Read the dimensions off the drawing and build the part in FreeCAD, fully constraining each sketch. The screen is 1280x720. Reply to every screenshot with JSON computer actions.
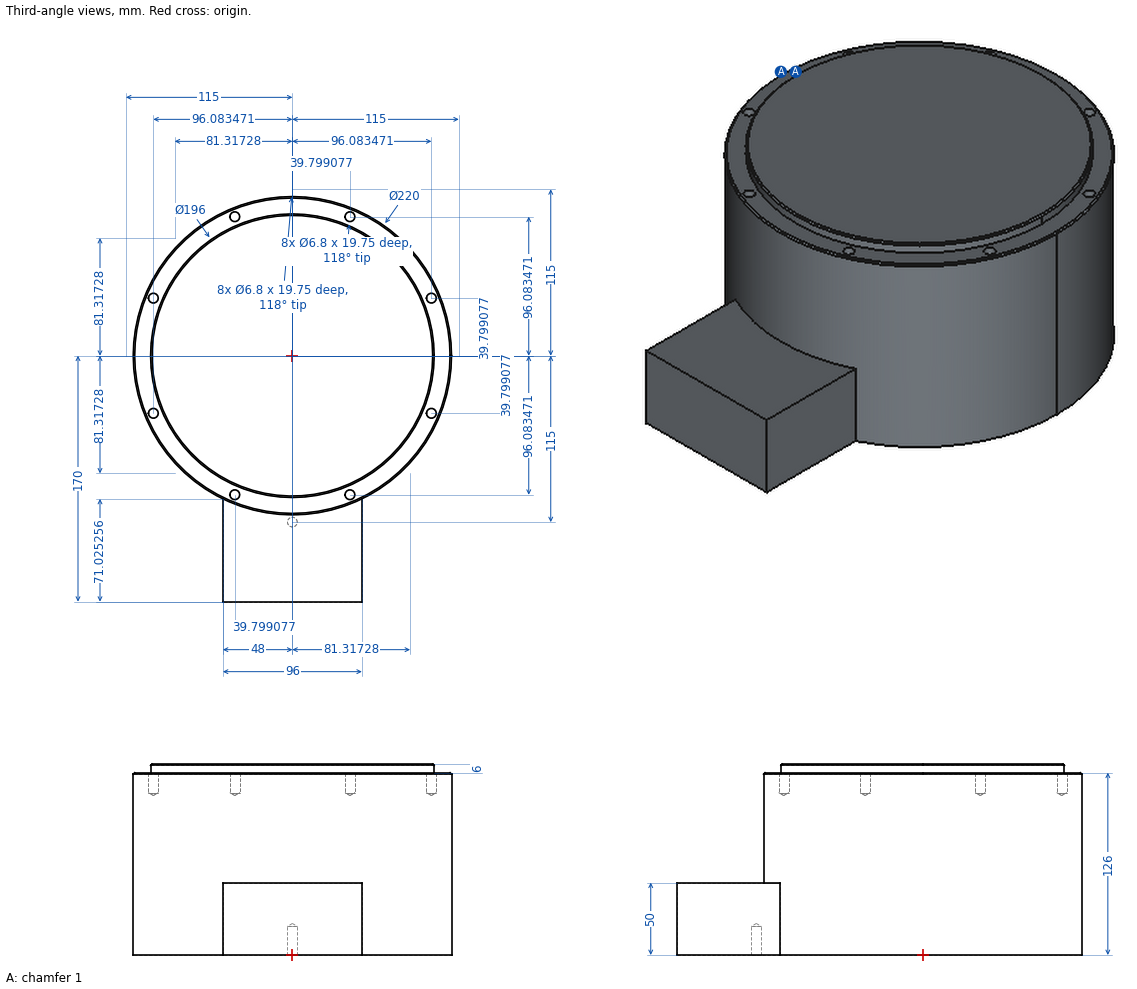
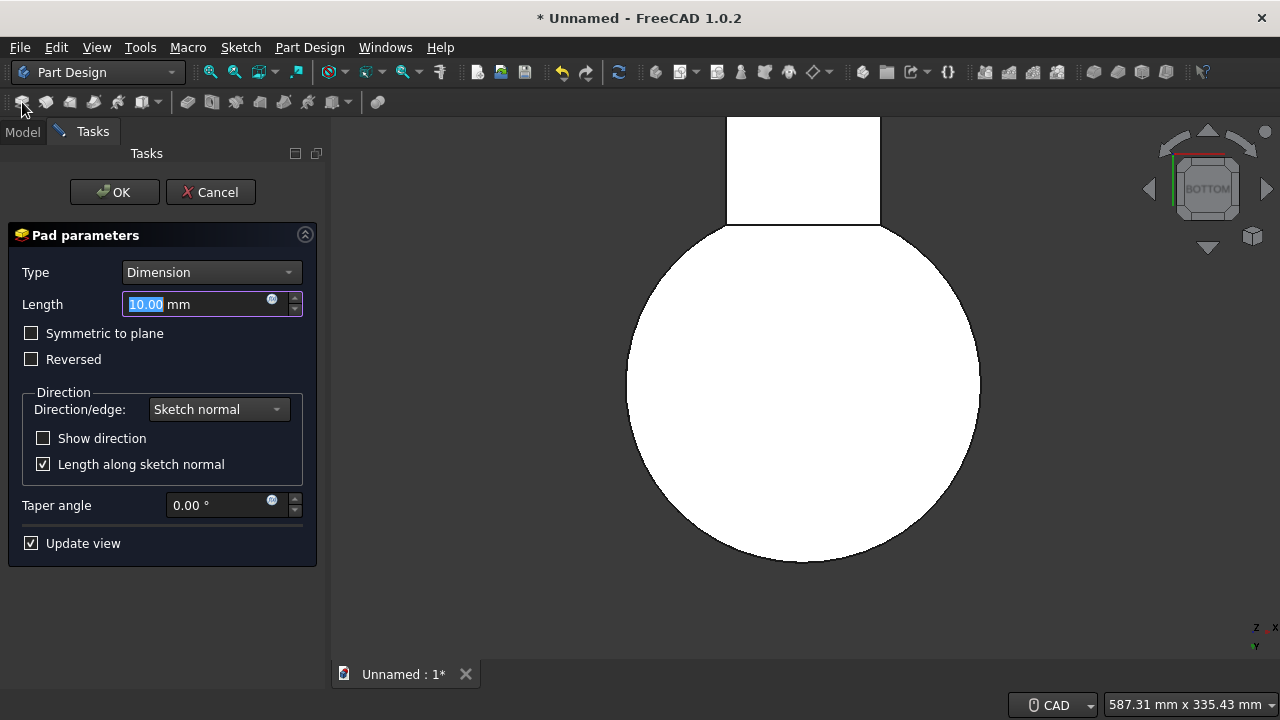
{"action": "type", "text": "50"}
{"action": "key", "text": "Tab"}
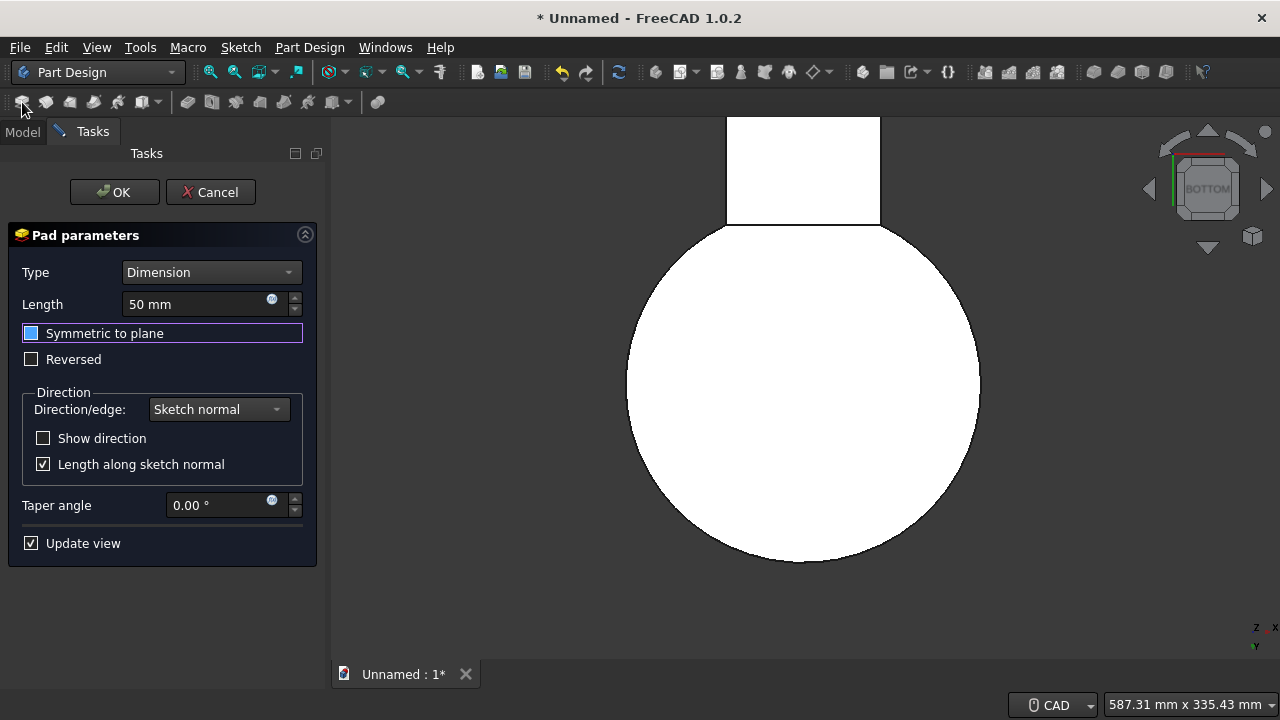
{"action": "left_click", "coordinate": [30, 359]}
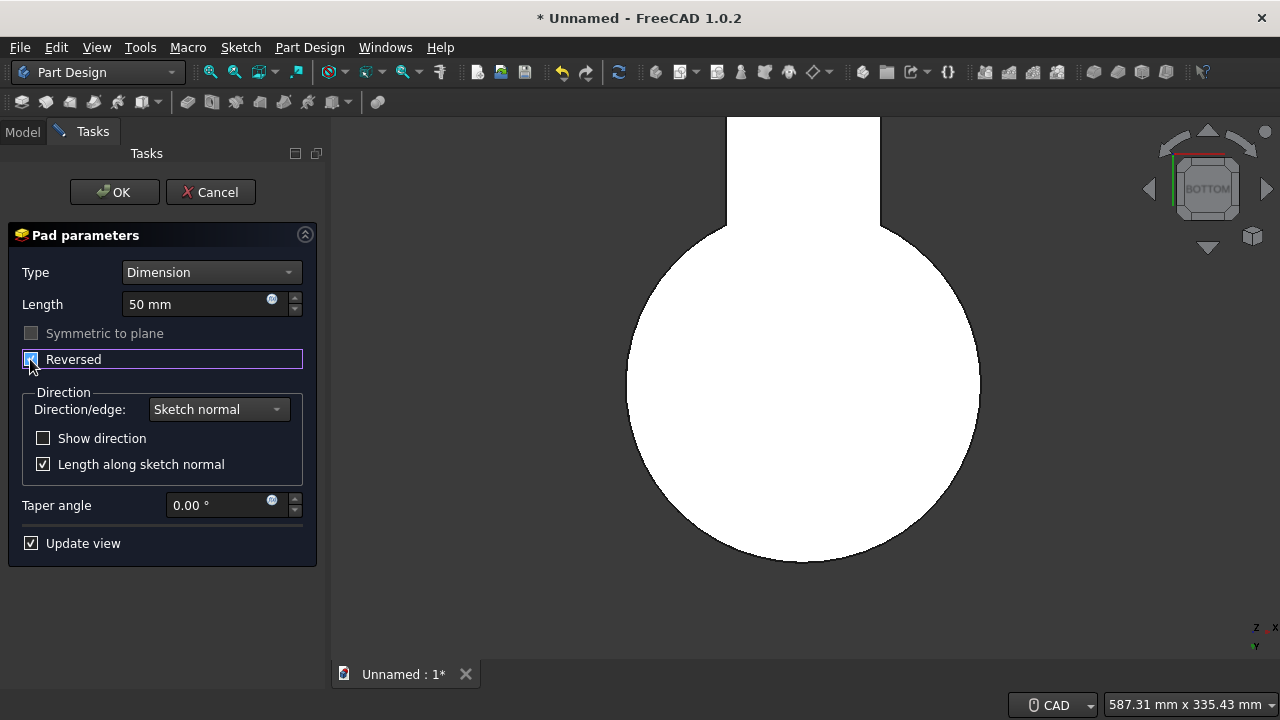
{"action": "left_click", "coordinate": [115, 192]}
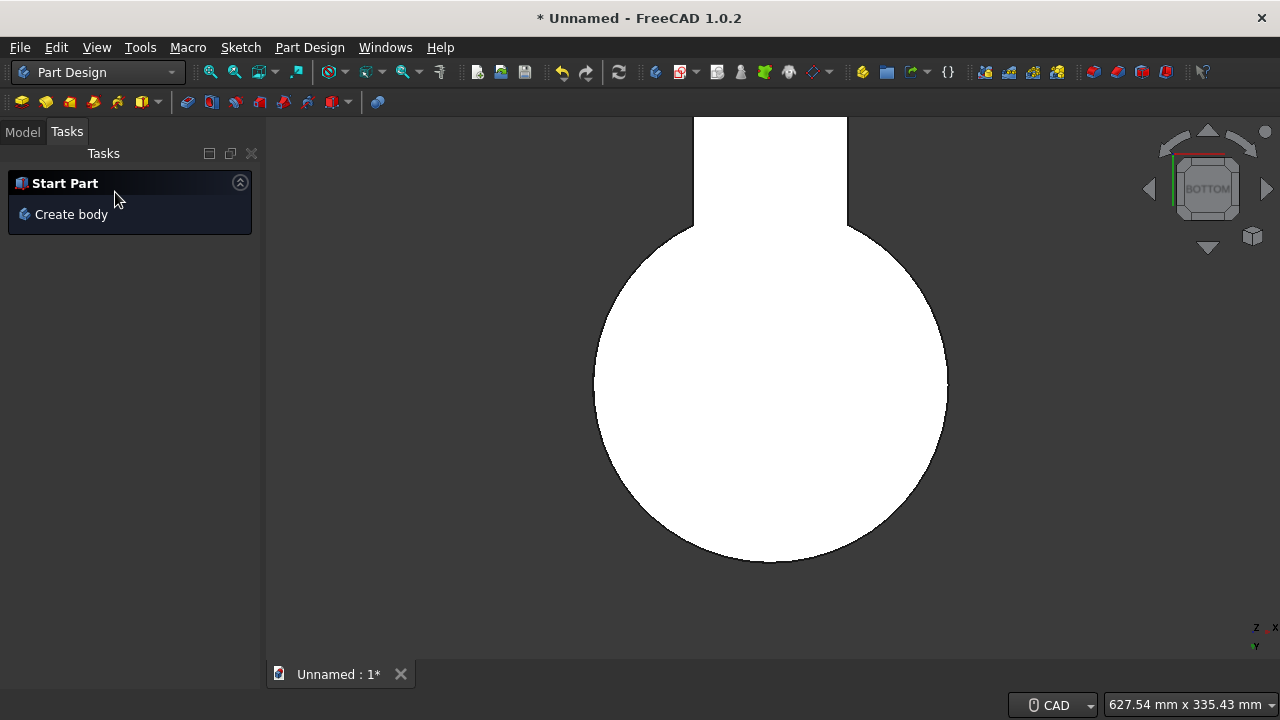
{"action": "left_click", "coordinate": [212, 72]}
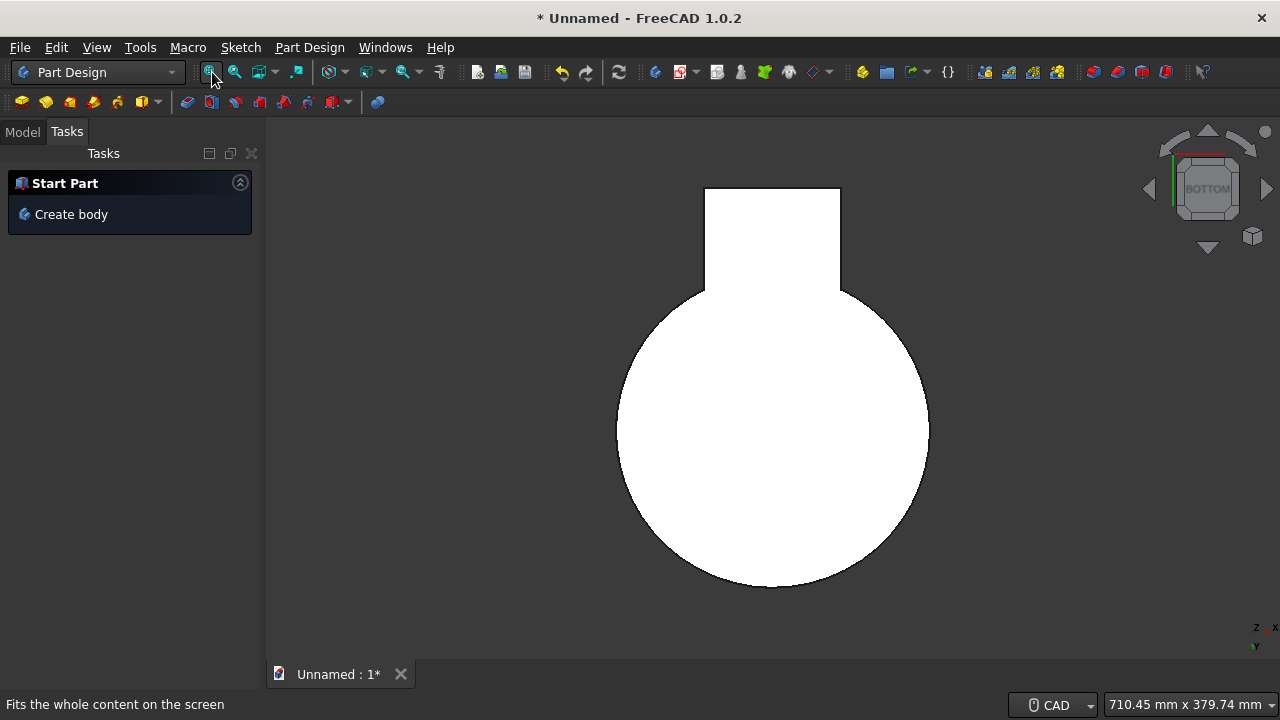
{"action": "key", "text": "0"}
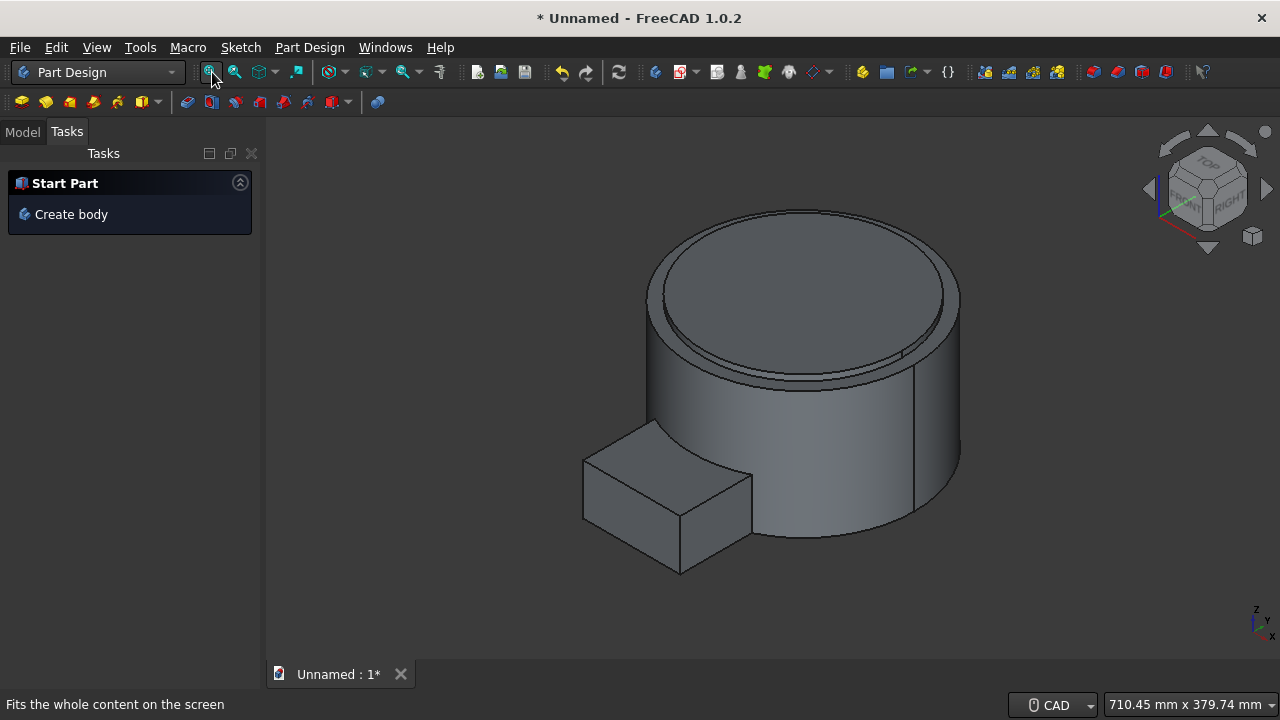
{"action": "left_click", "coordinate": [663, 341]}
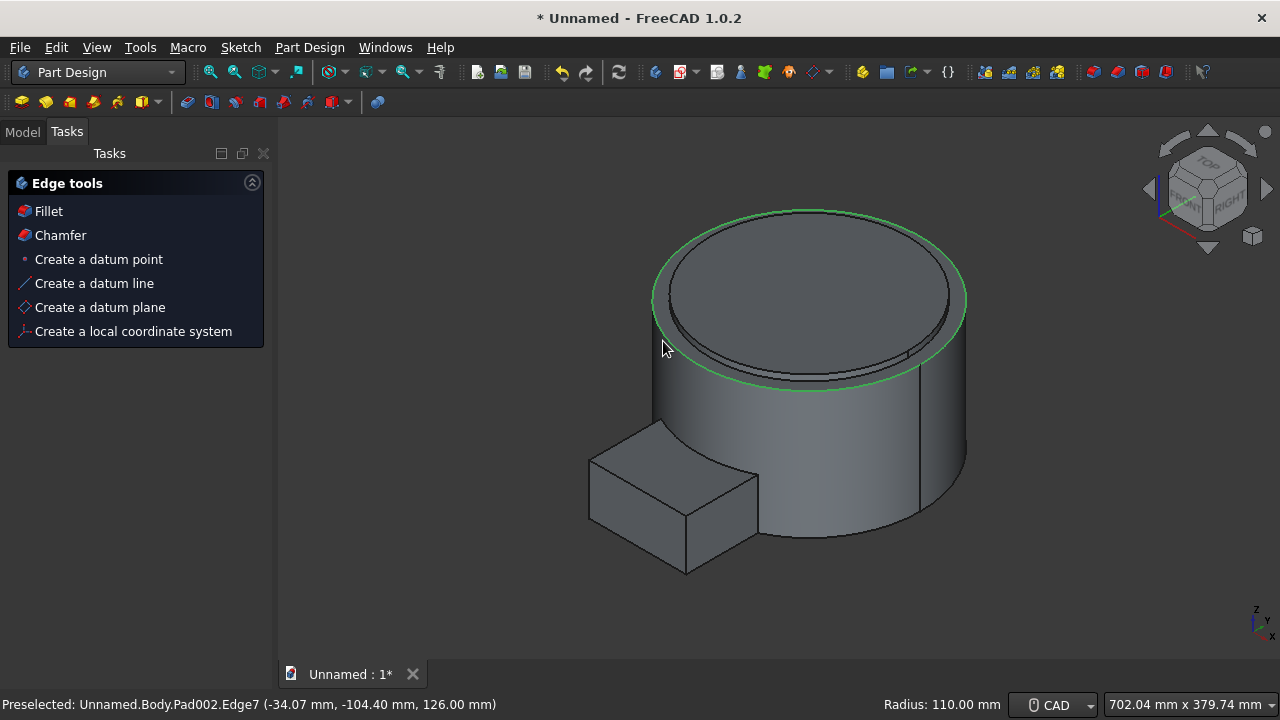
{"action": "left_click", "coordinate": [685, 329], "text": "ctrl"}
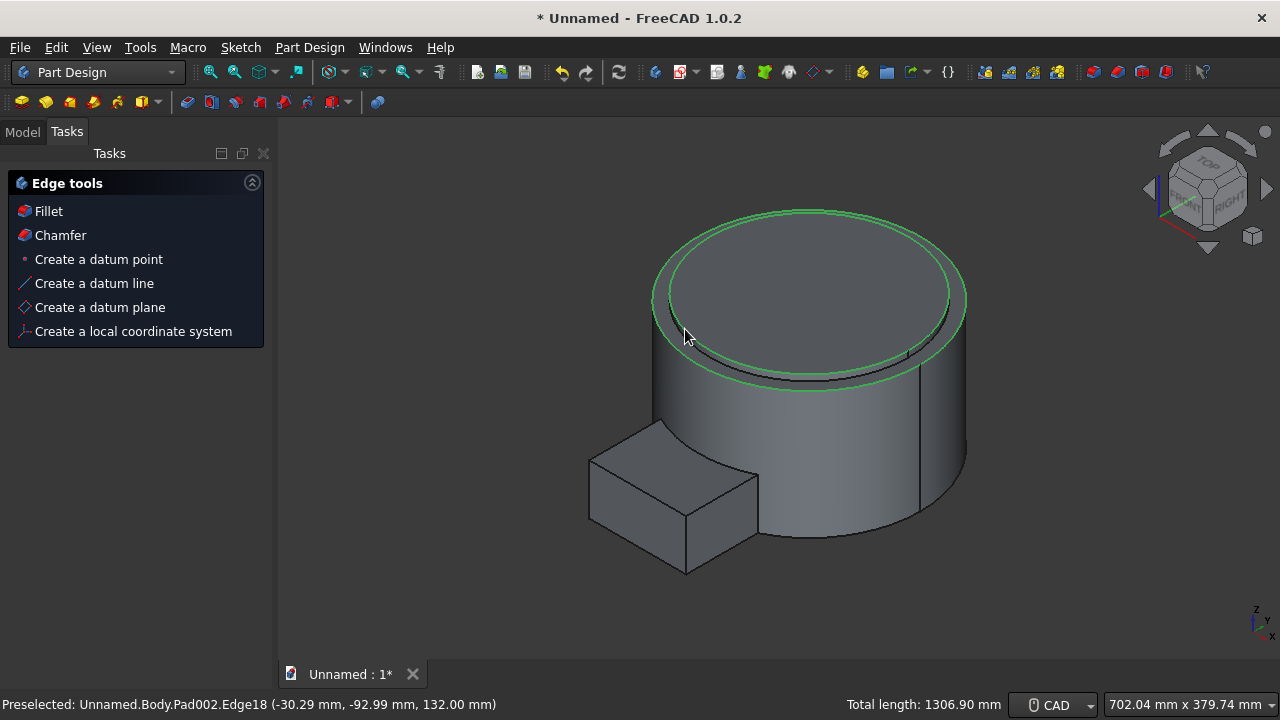
{"action": "left_click", "coordinate": [1118, 72]}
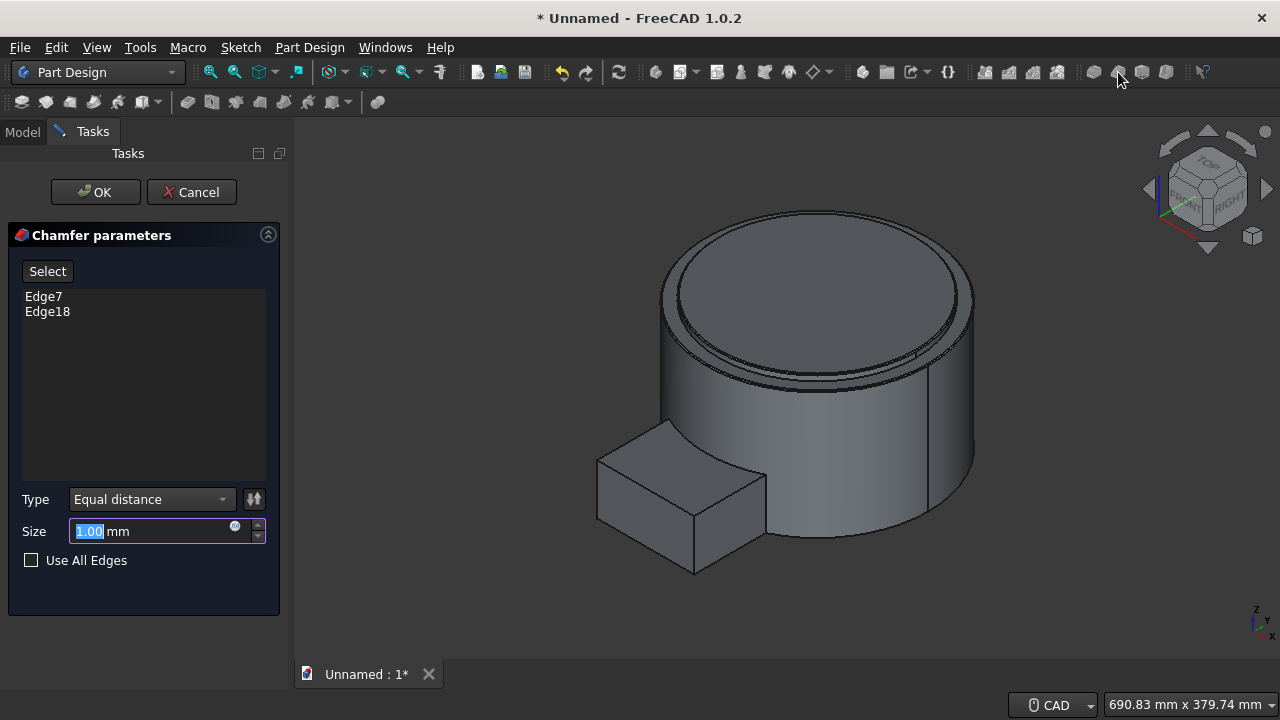
{"action": "type", "text": "1"}
{"action": "key", "text": "Tab"}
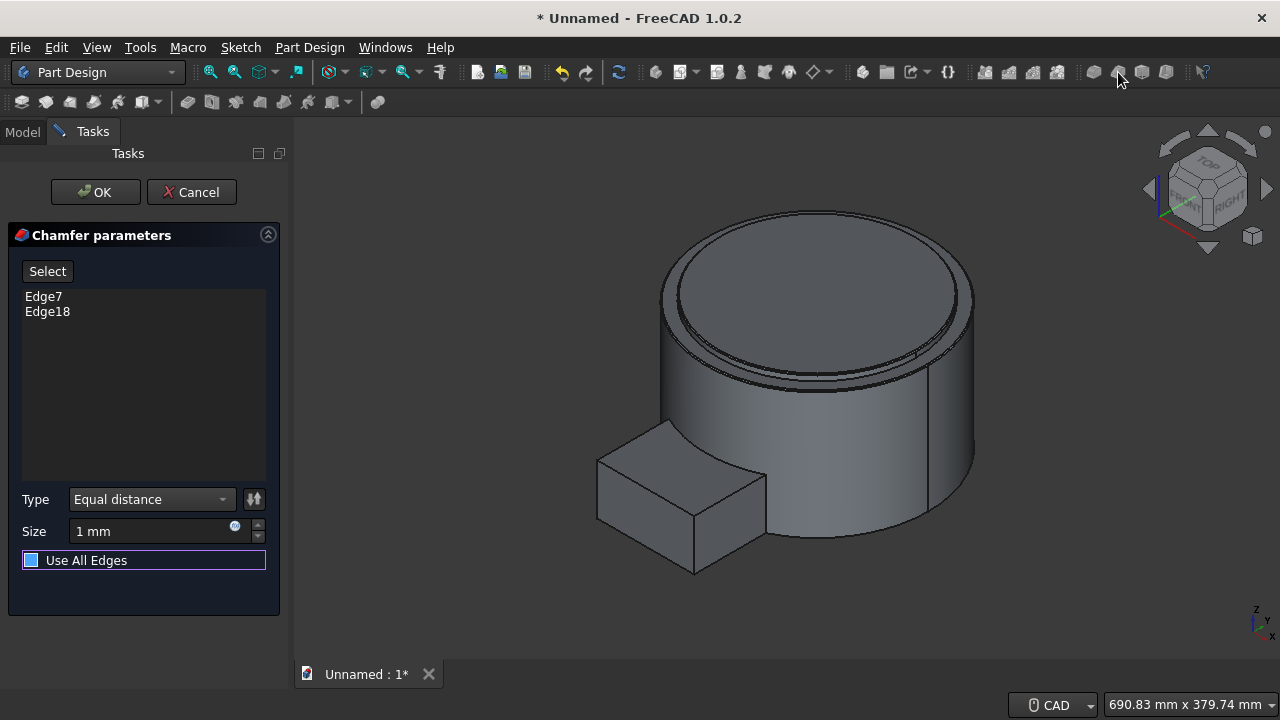
{"action": "left_click", "coordinate": [96, 192]}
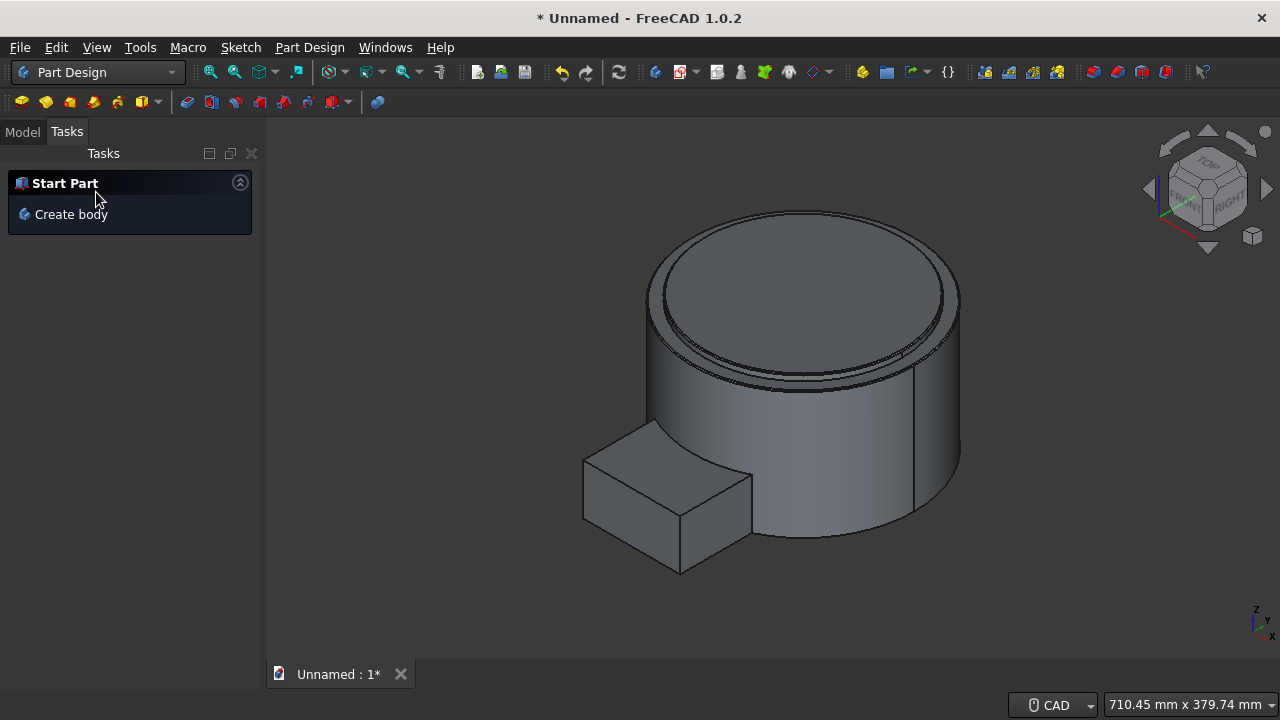
{"action": "key", "text": "5"}